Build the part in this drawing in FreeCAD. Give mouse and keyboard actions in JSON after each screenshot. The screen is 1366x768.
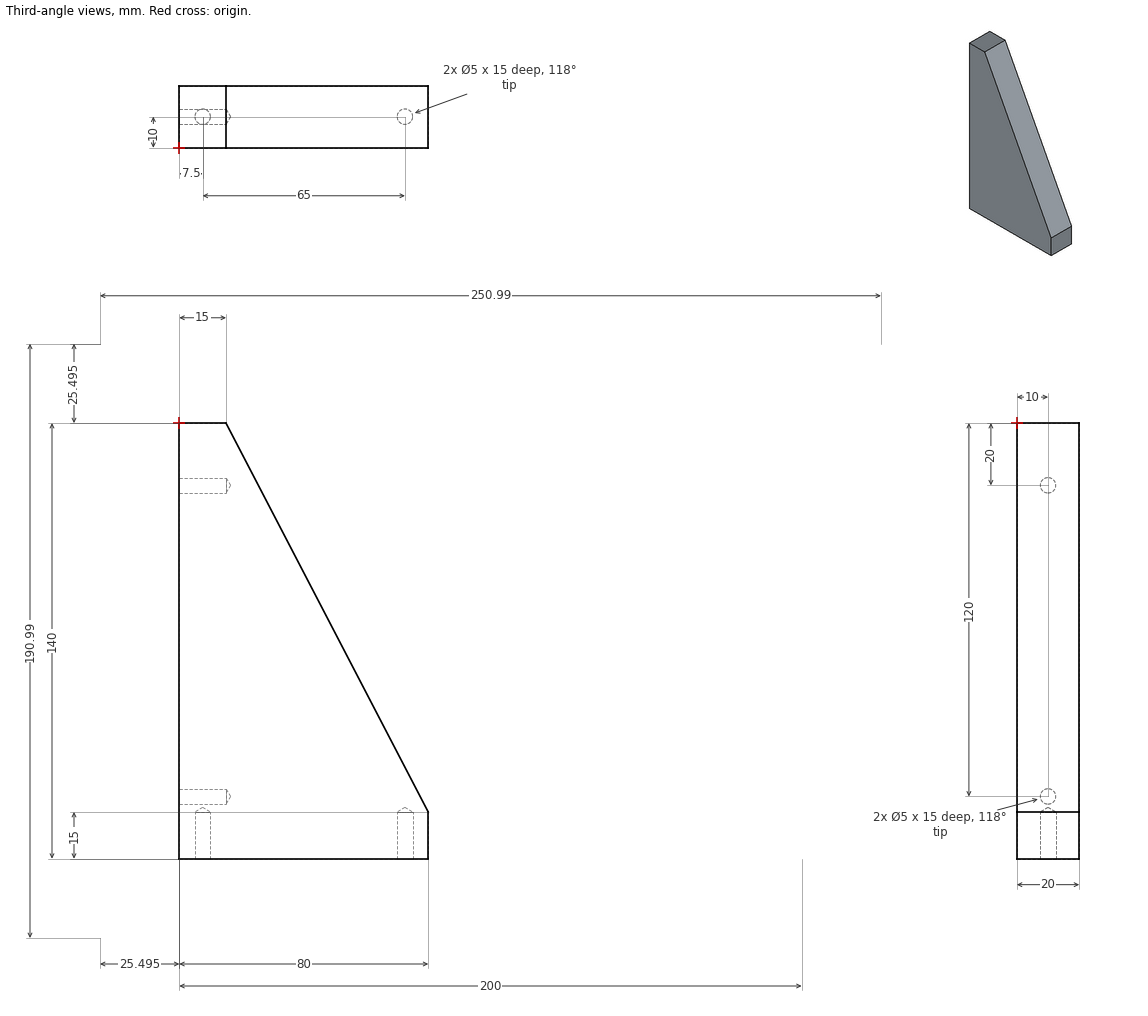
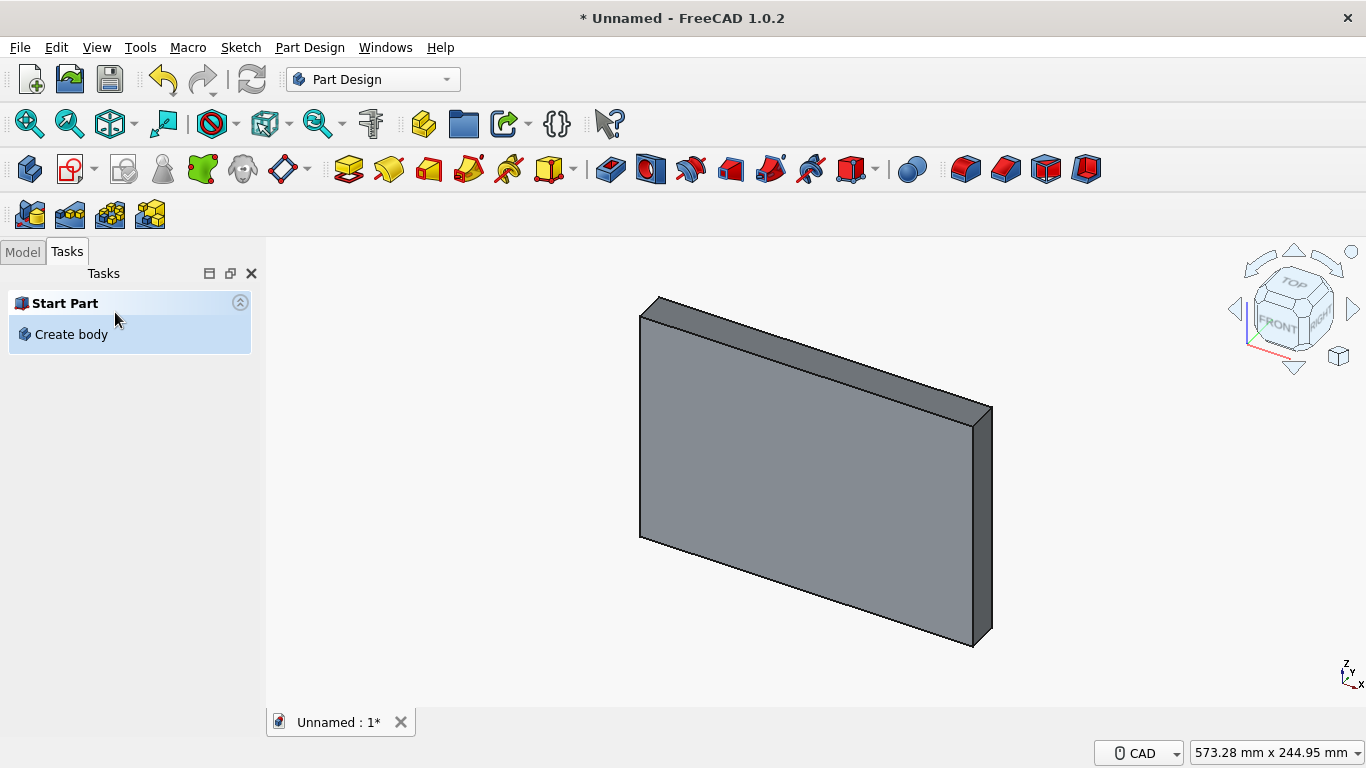
{"action": "key", "text": "4"}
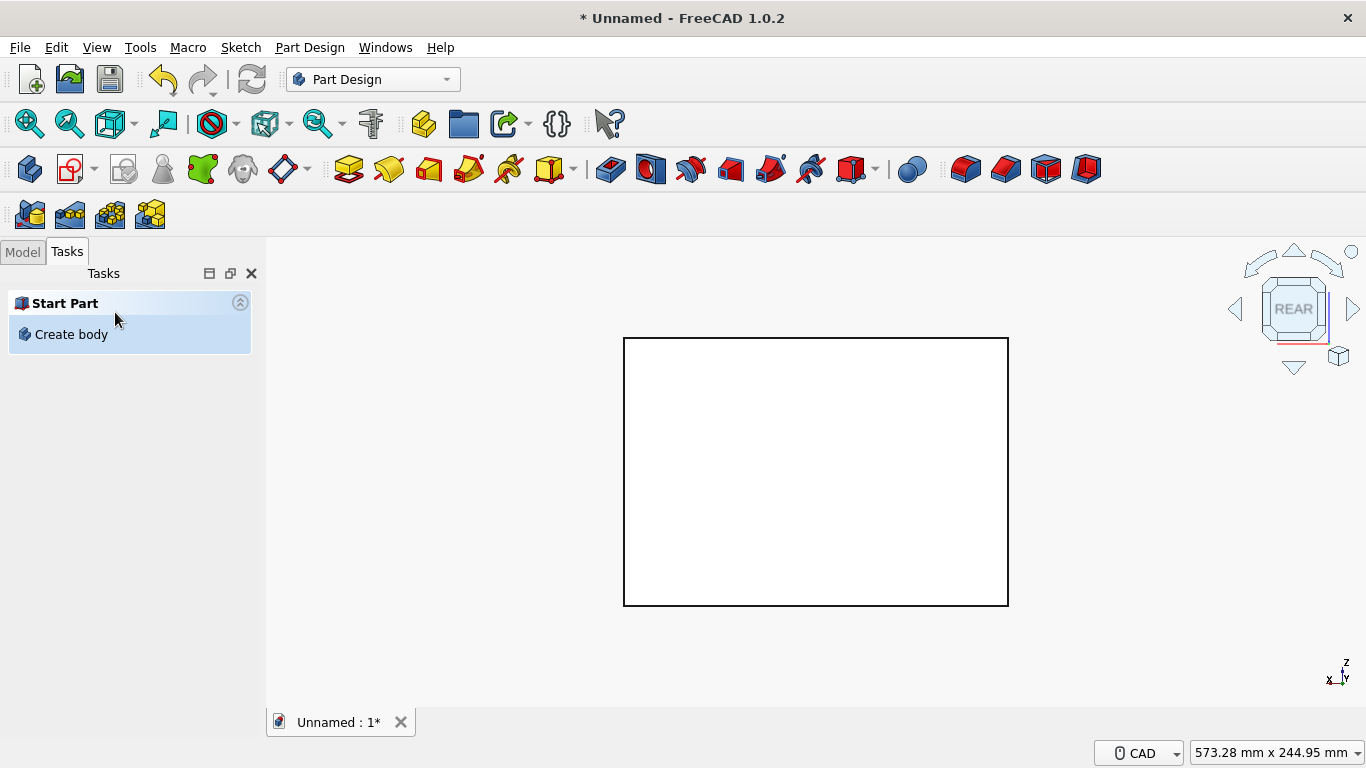
{"action": "left_click", "coordinate": [761, 471]}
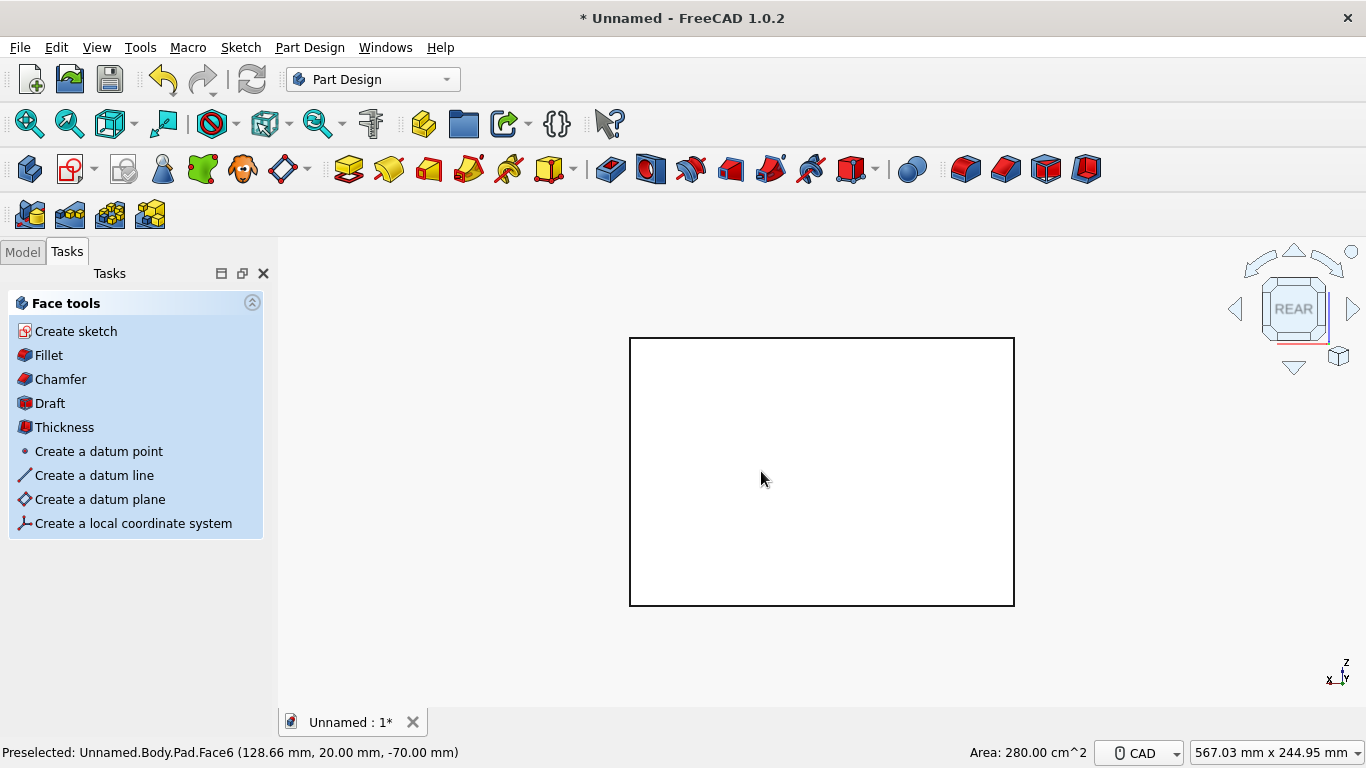
{"action": "left_click", "coordinate": [70, 170]}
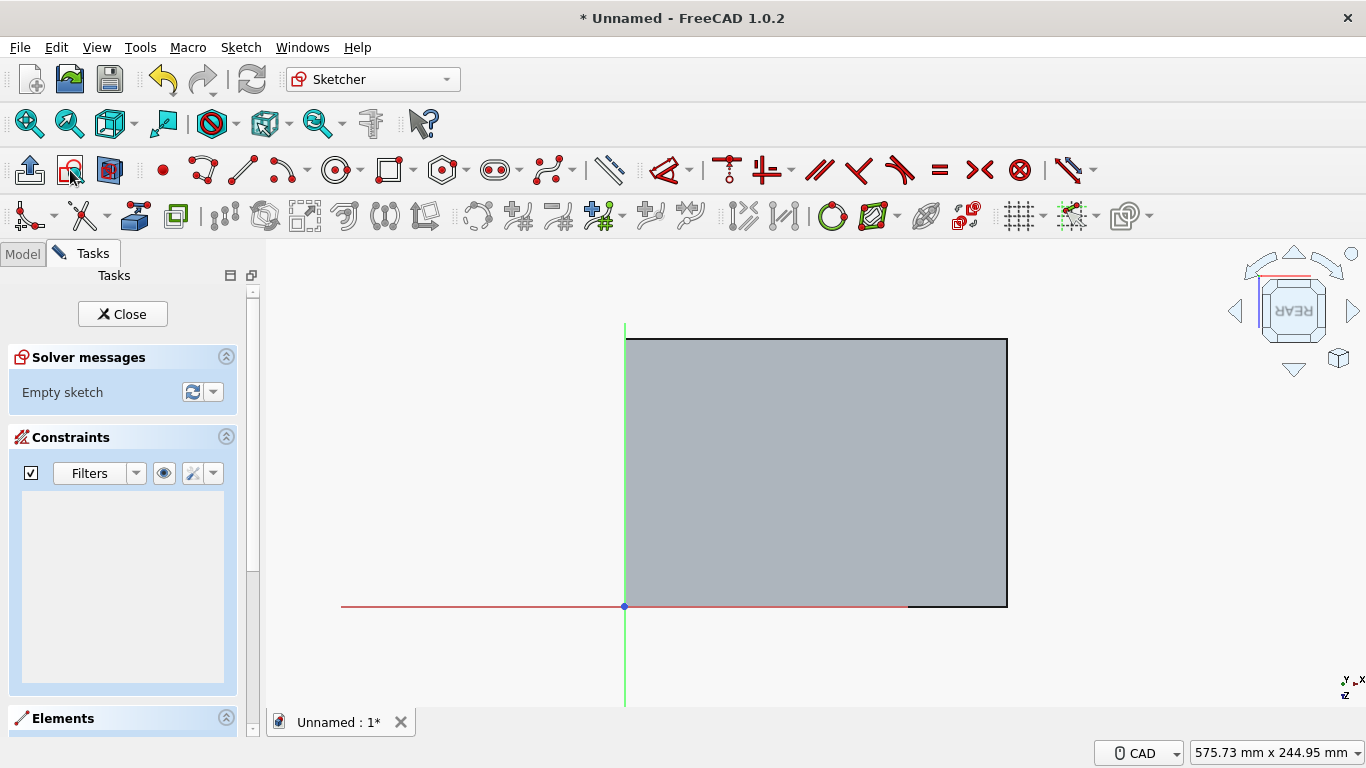
{"action": "scroll", "coordinate": [438, 473], "scroll_direction": "down", "scroll_amount": 1}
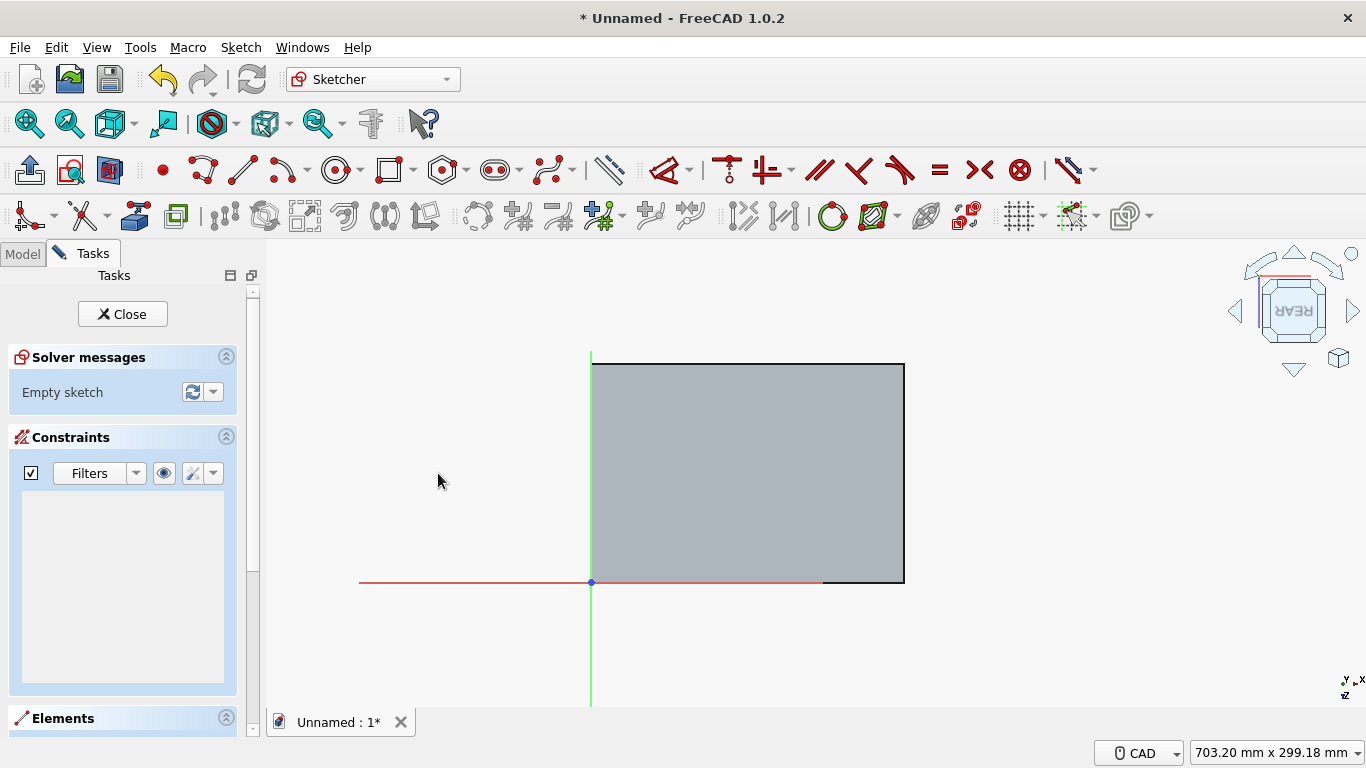
{"action": "key", "text": "g r"}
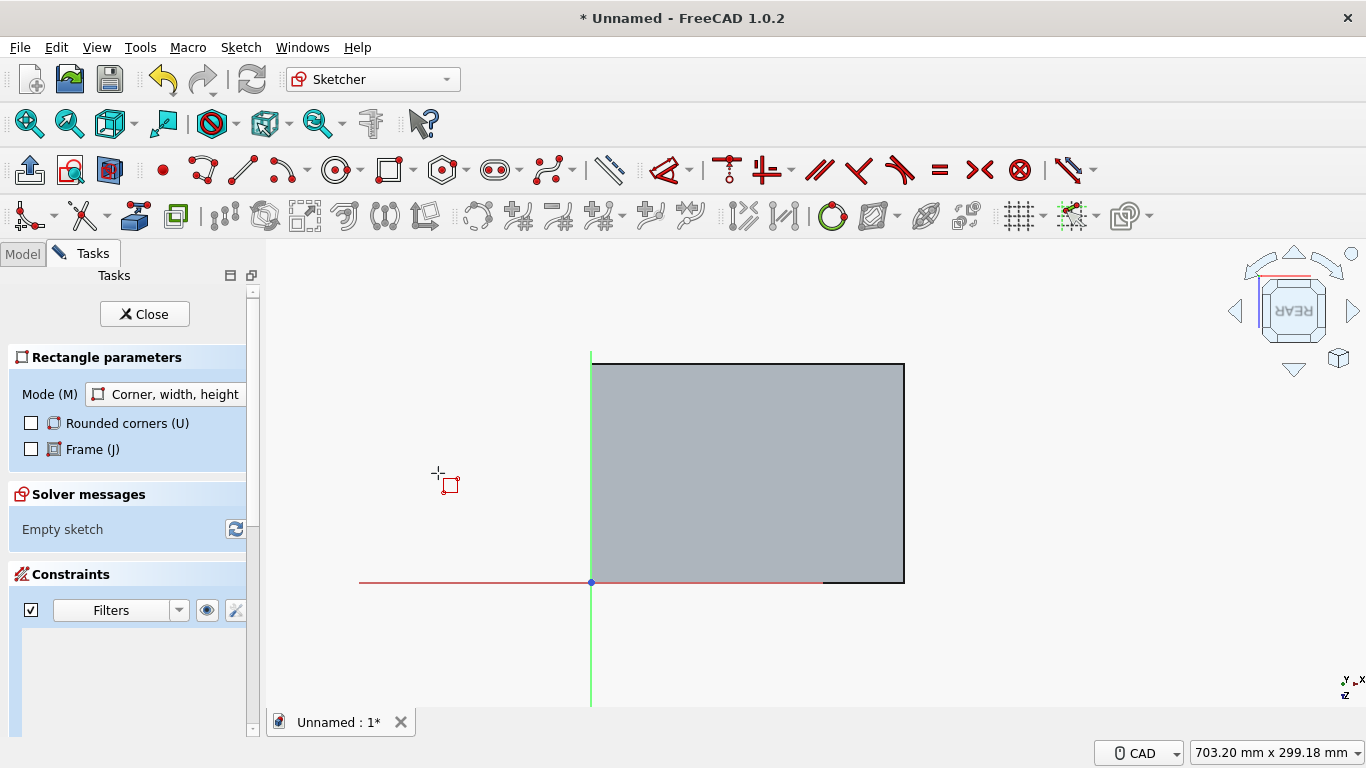
{"action": "left_click", "coordinate": [551, 324]}
{"action": "left_click", "coordinate": [944, 622]}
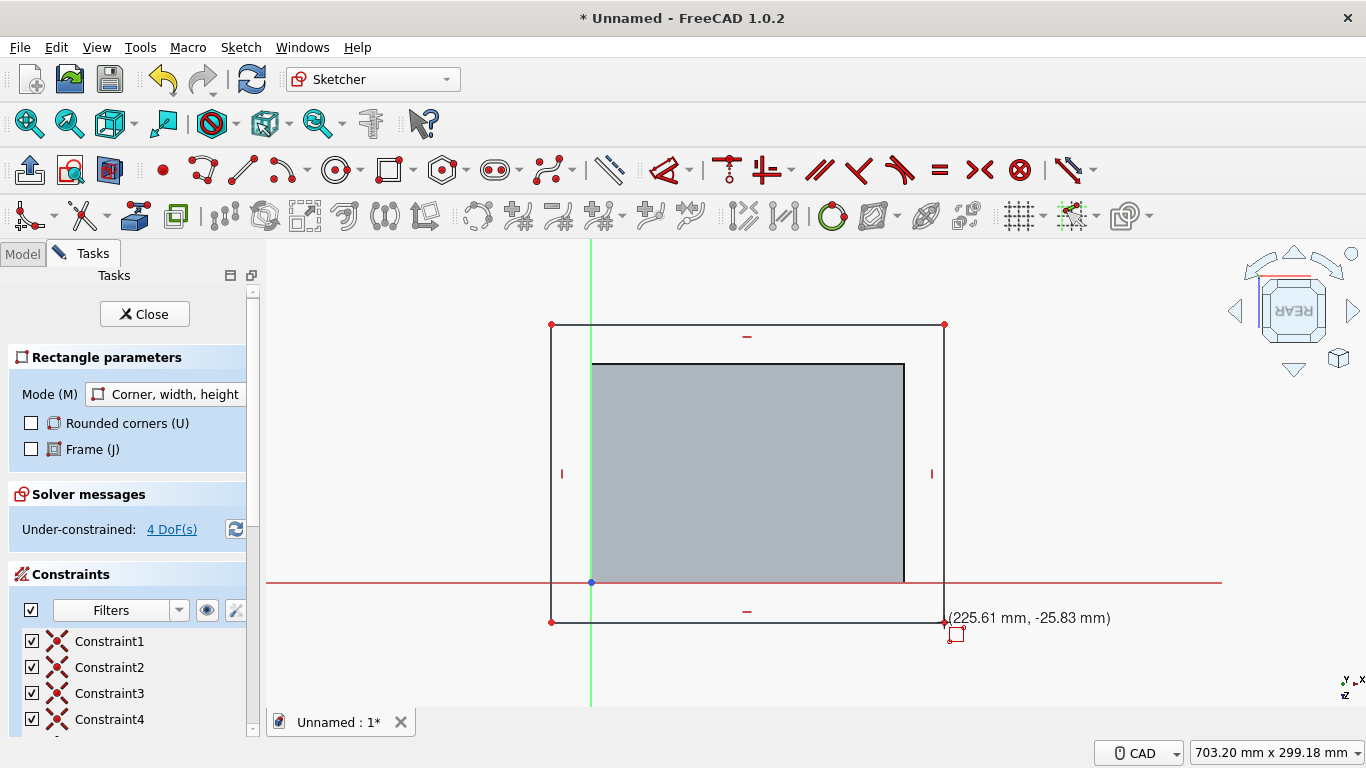
{"action": "key", "text": "g m"}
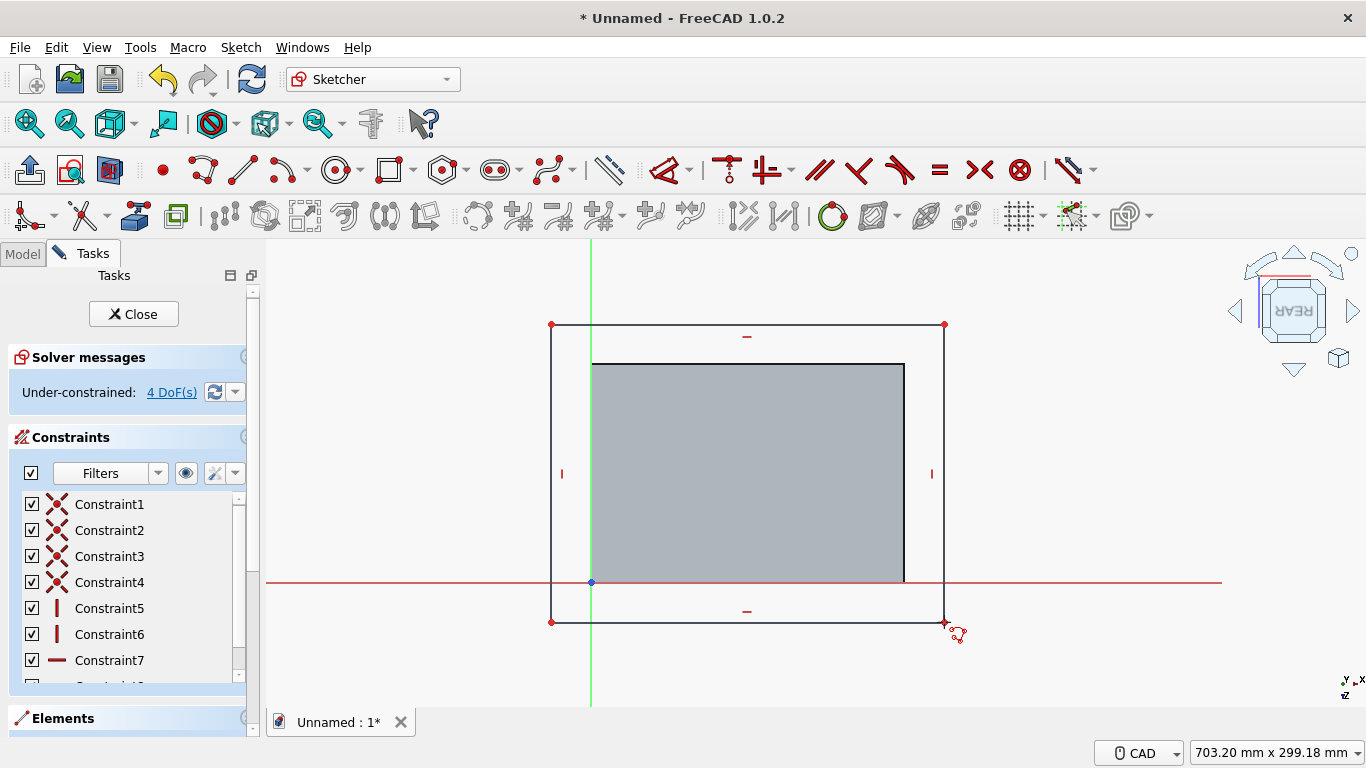
{"action": "left_click", "coordinate": [591, 583]}
{"action": "left_click", "coordinate": [600, 364]}
{"action": "left_click", "coordinate": [716, 364]}
{"action": "left_click", "coordinate": [716, 387]}
{"action": "left_click", "coordinate": [615, 574]}
{"action": "left_click", "coordinate": [591, 583]}
{"action": "key", "text": "Escape"}
{"action": "key", "text": "Escape"}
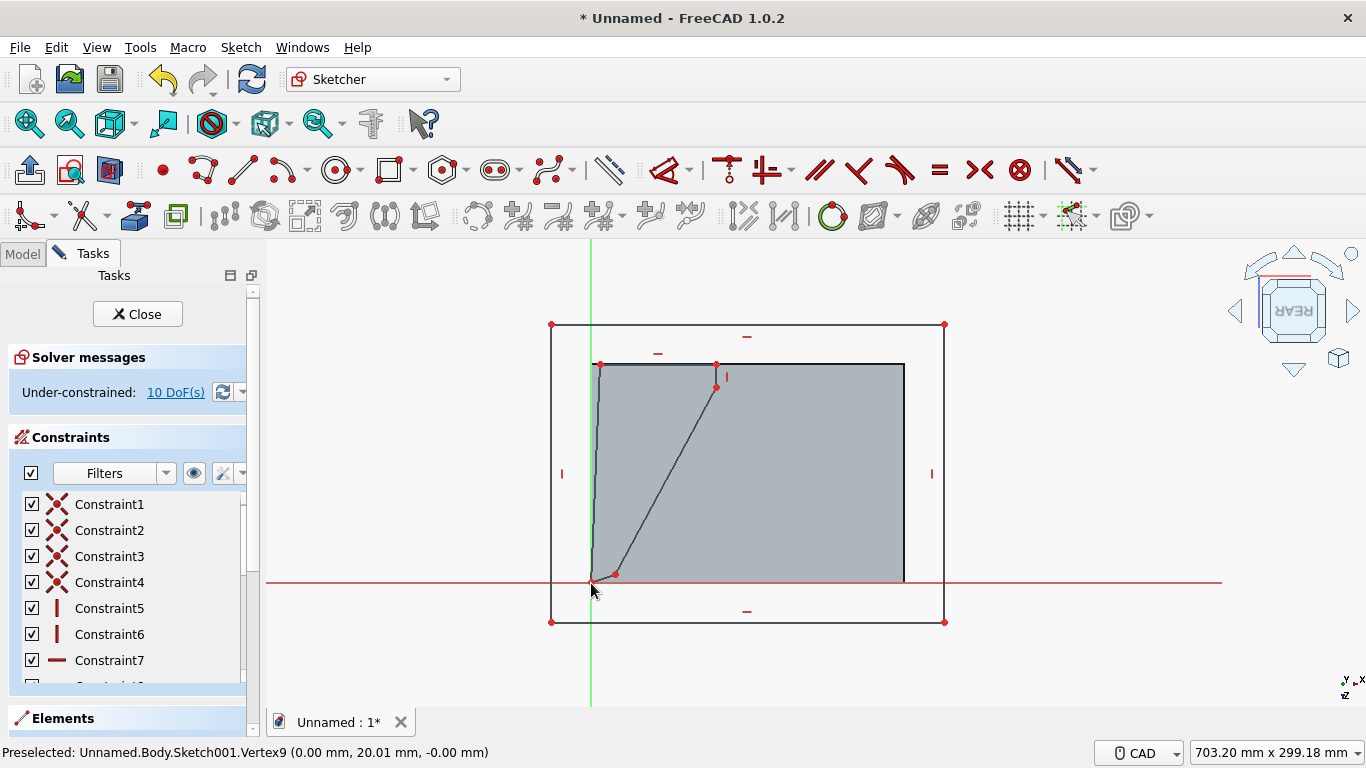
{"action": "left_click", "coordinate": [594, 517]}